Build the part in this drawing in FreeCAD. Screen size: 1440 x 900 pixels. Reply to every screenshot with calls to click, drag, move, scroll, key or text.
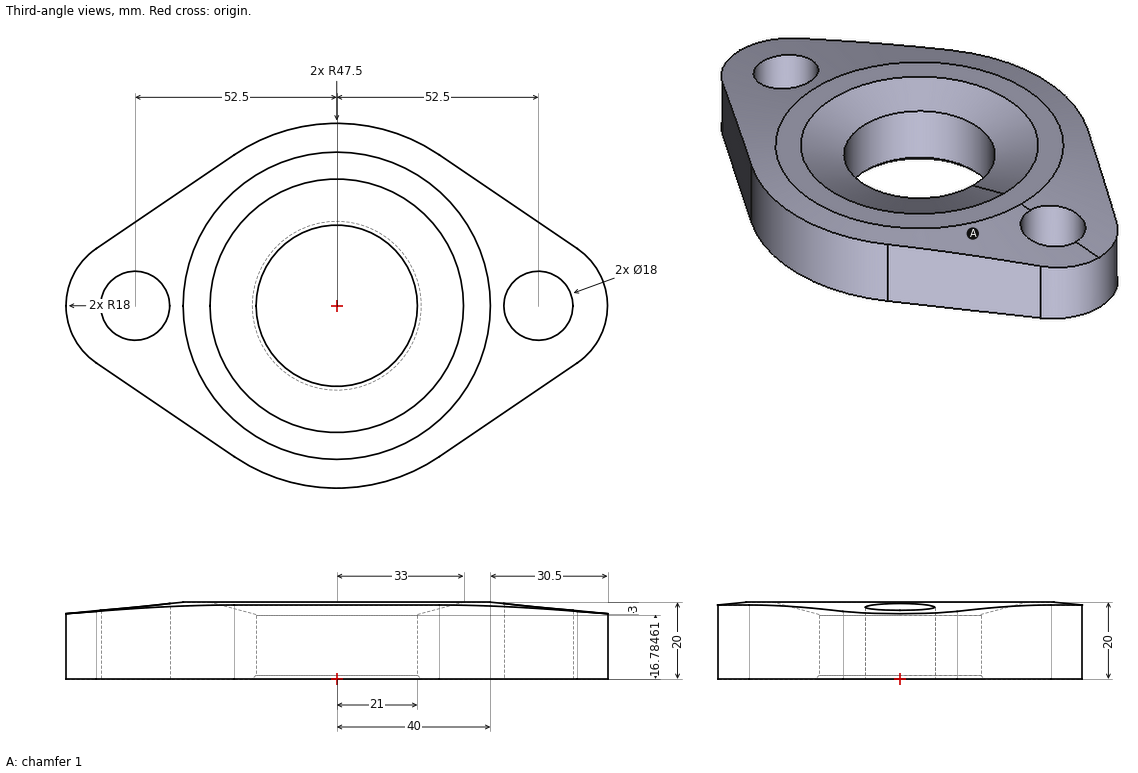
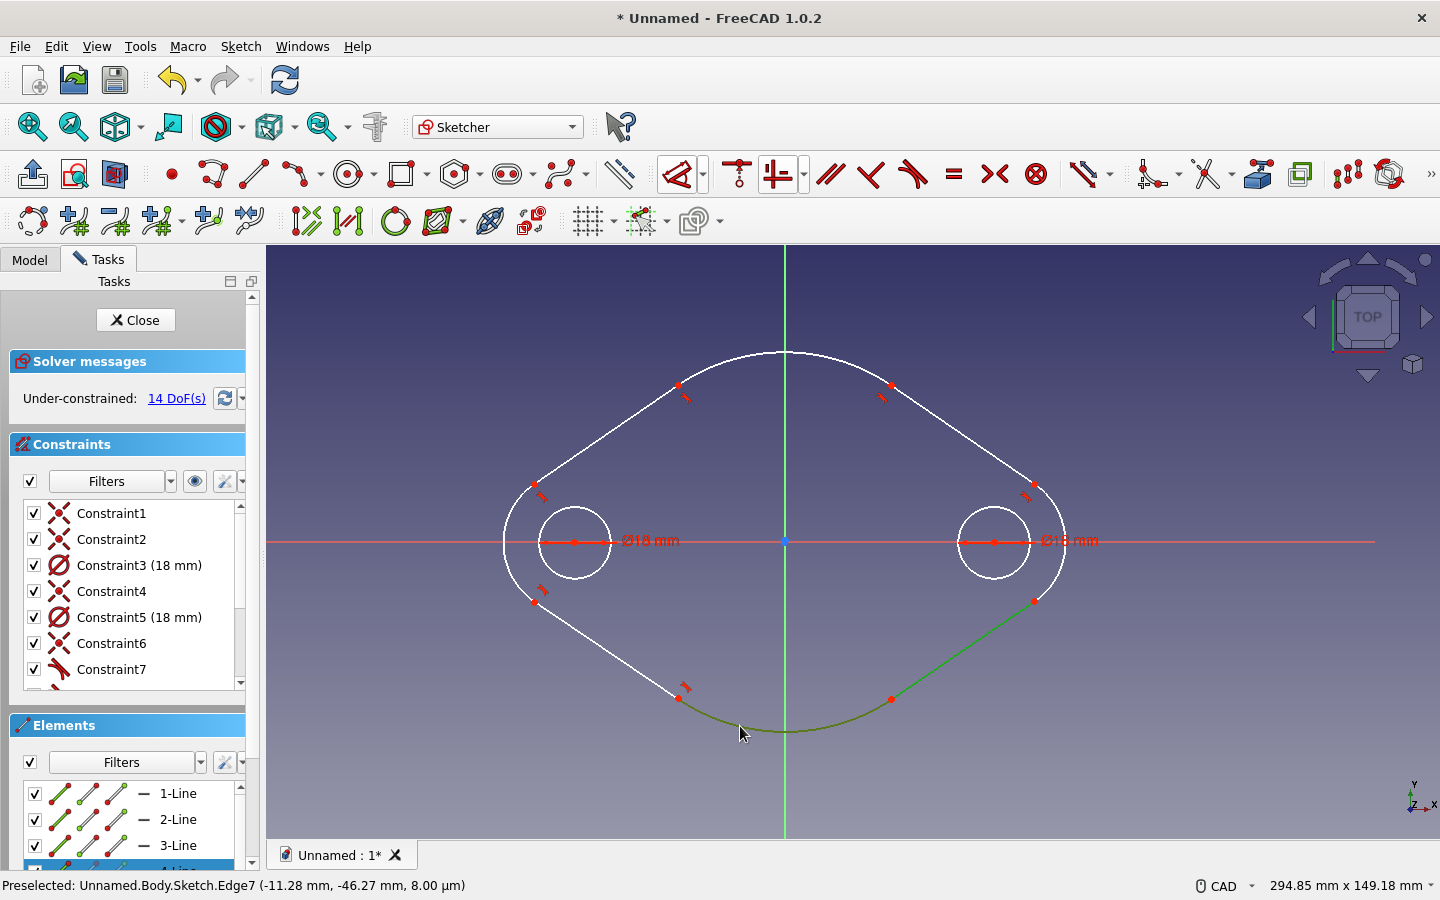
key(t)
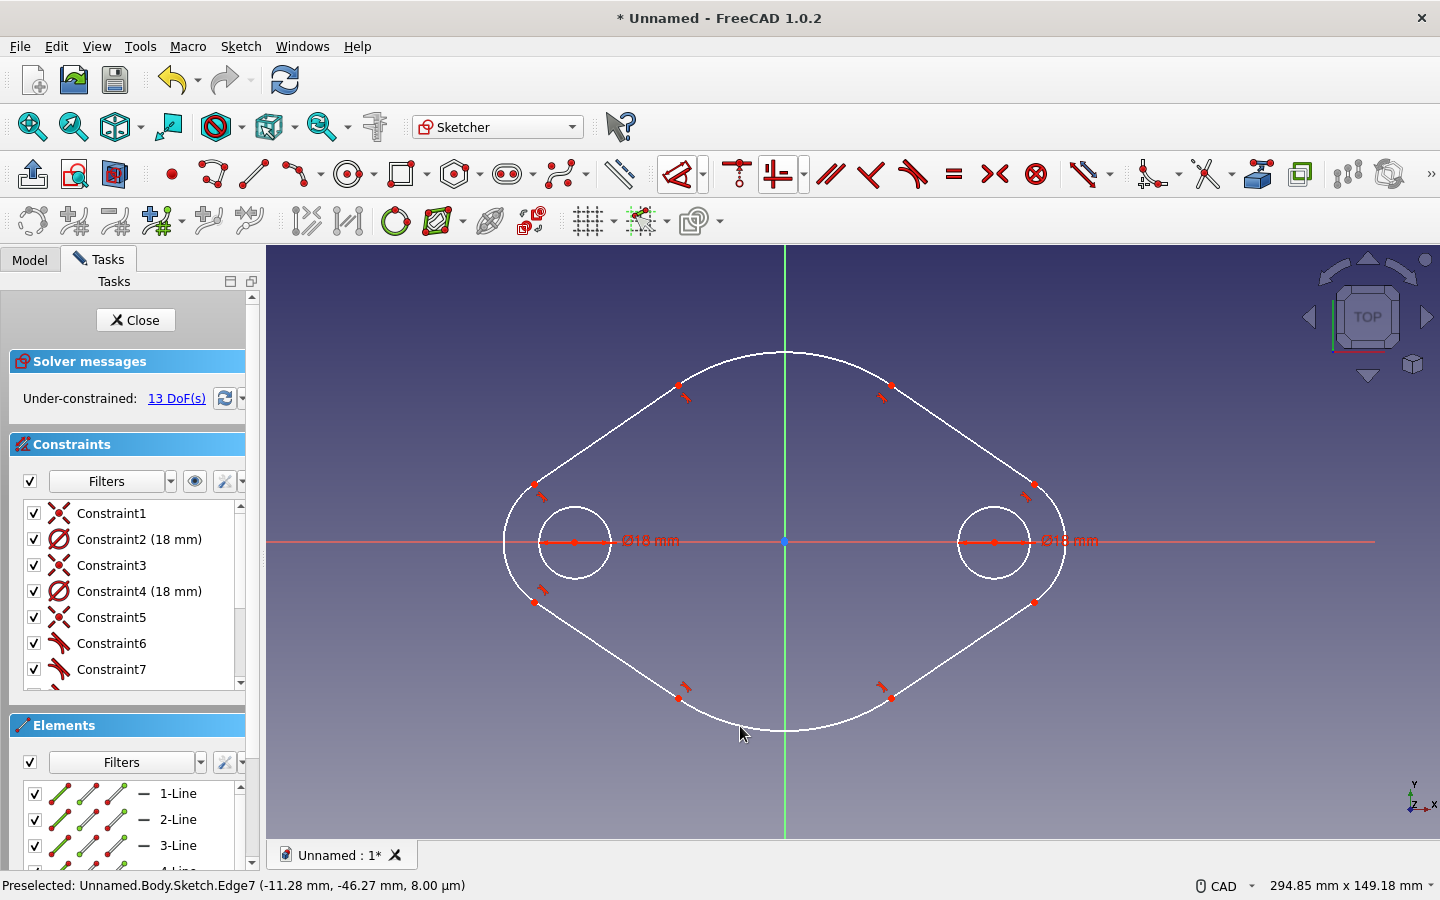
click(934, 670)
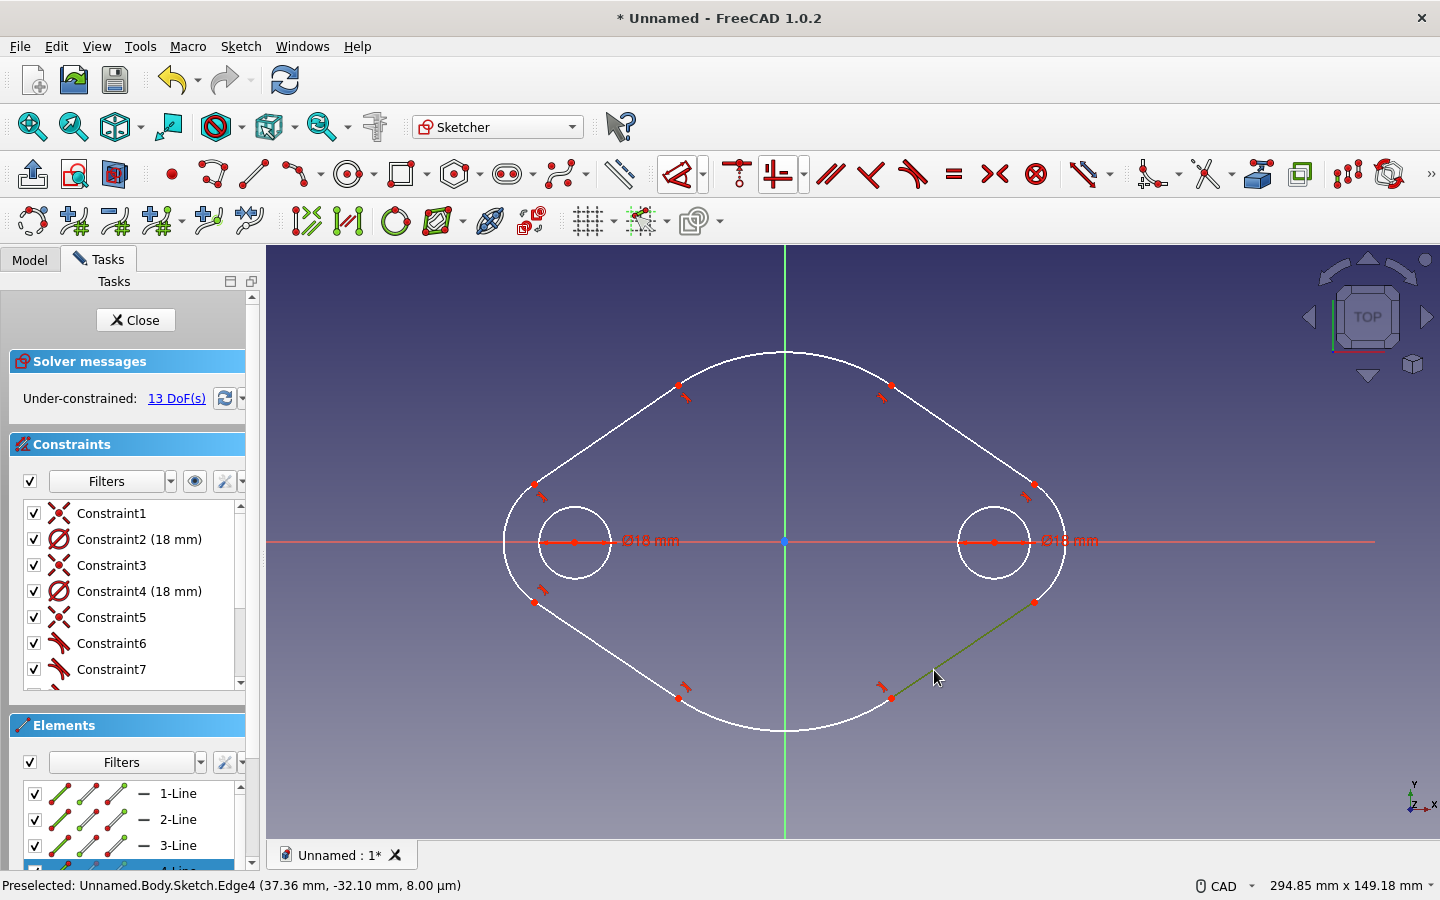
click(1060, 570)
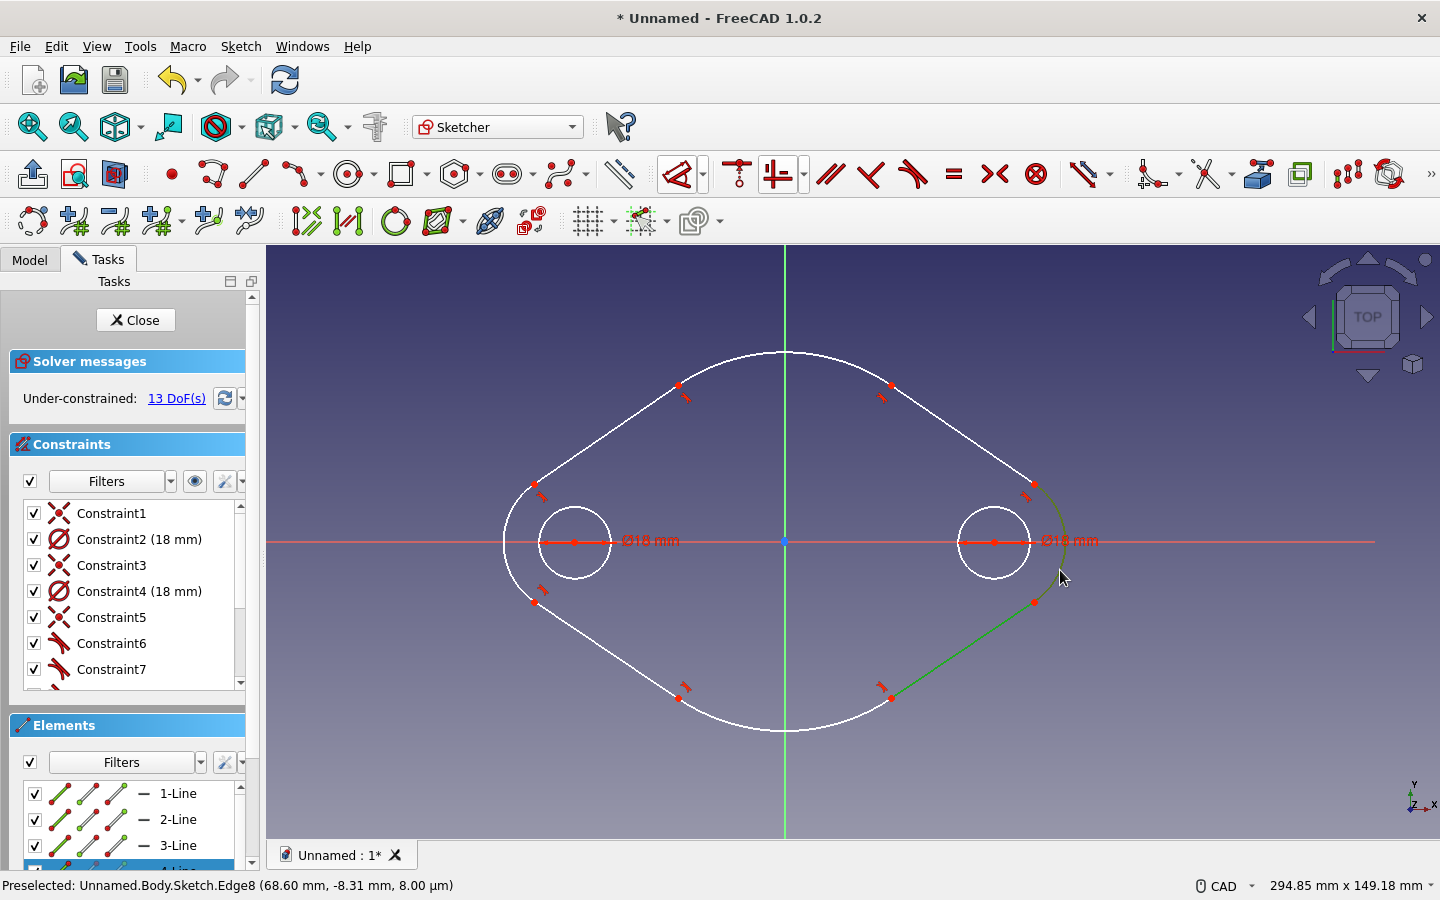
key(t)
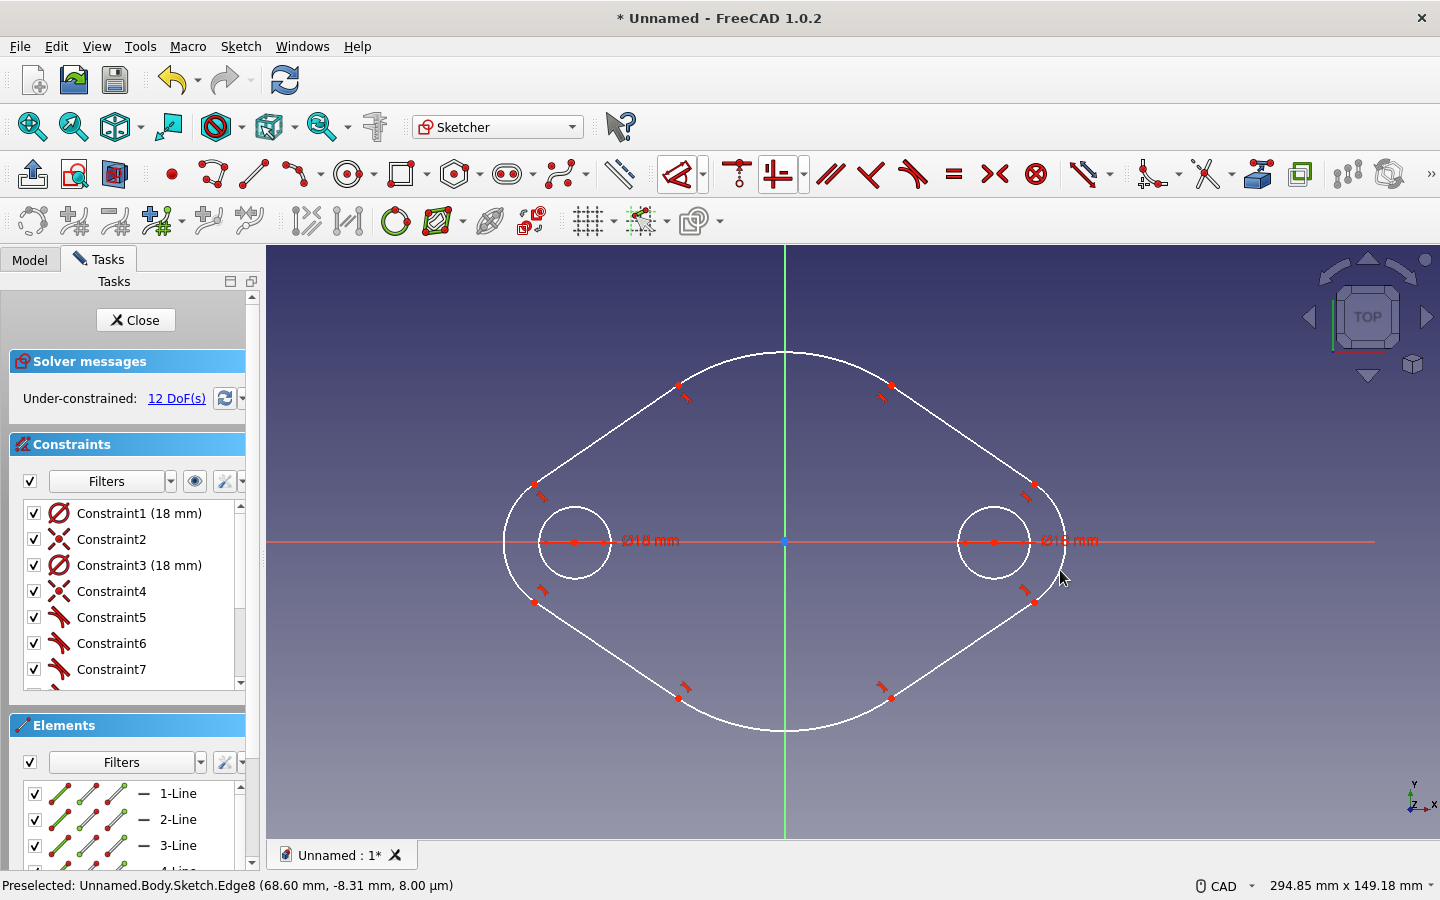
click(829, 358)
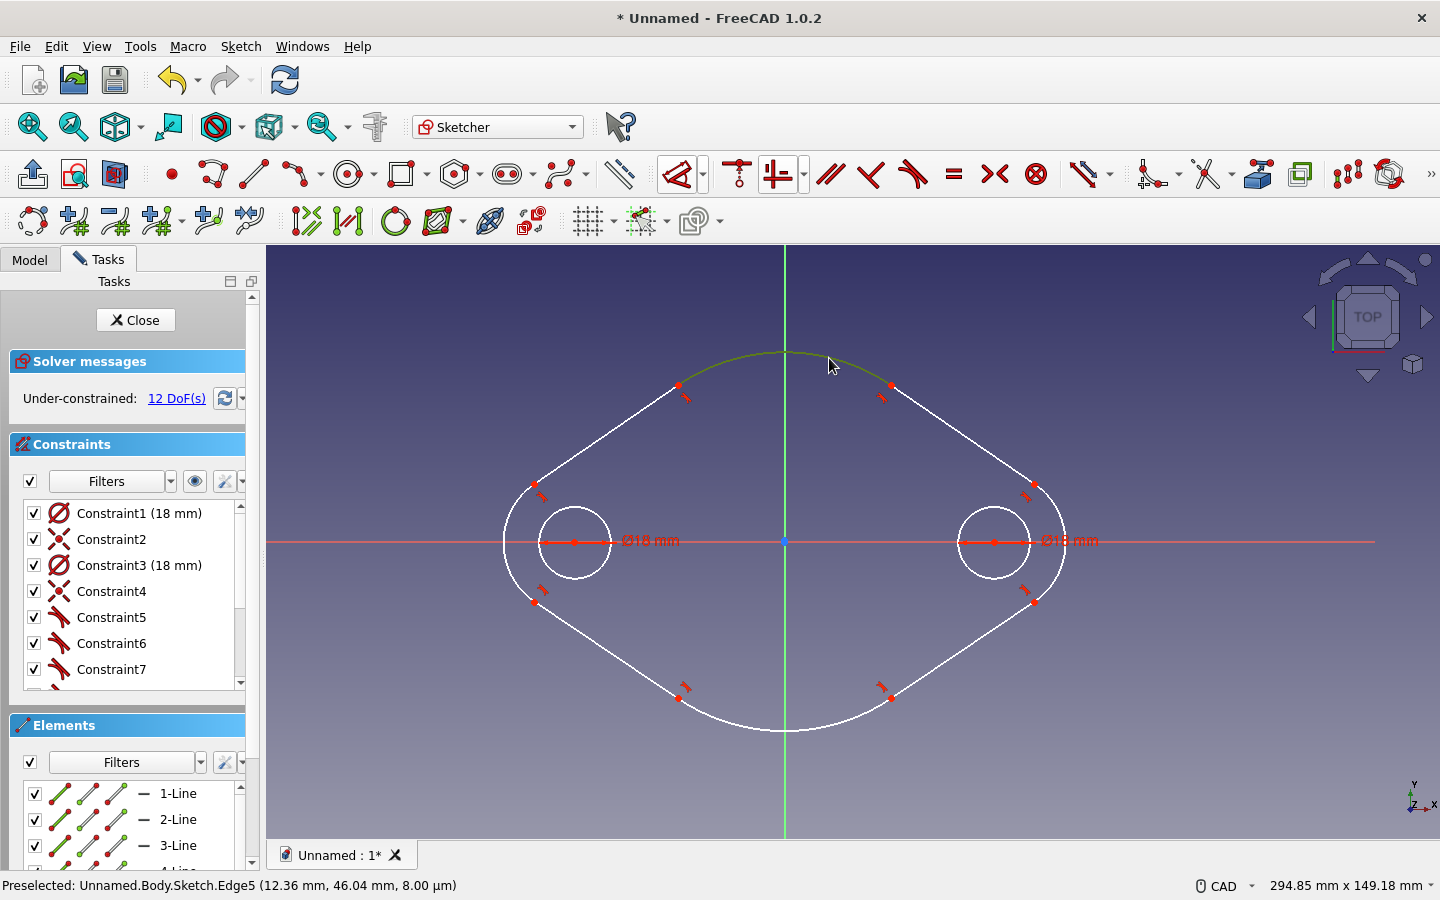
click(740, 726)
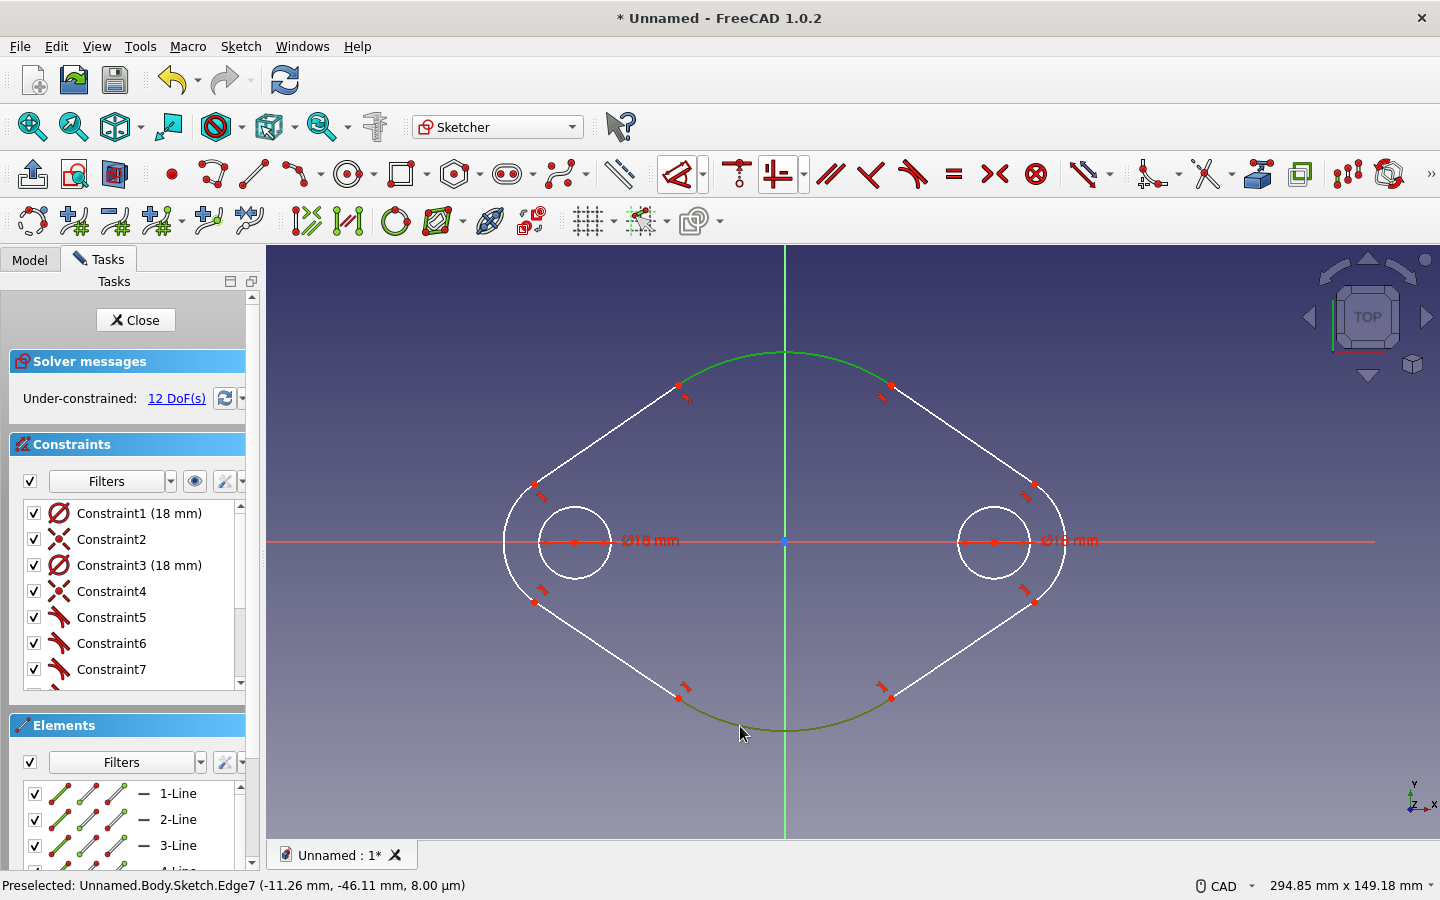
key(c)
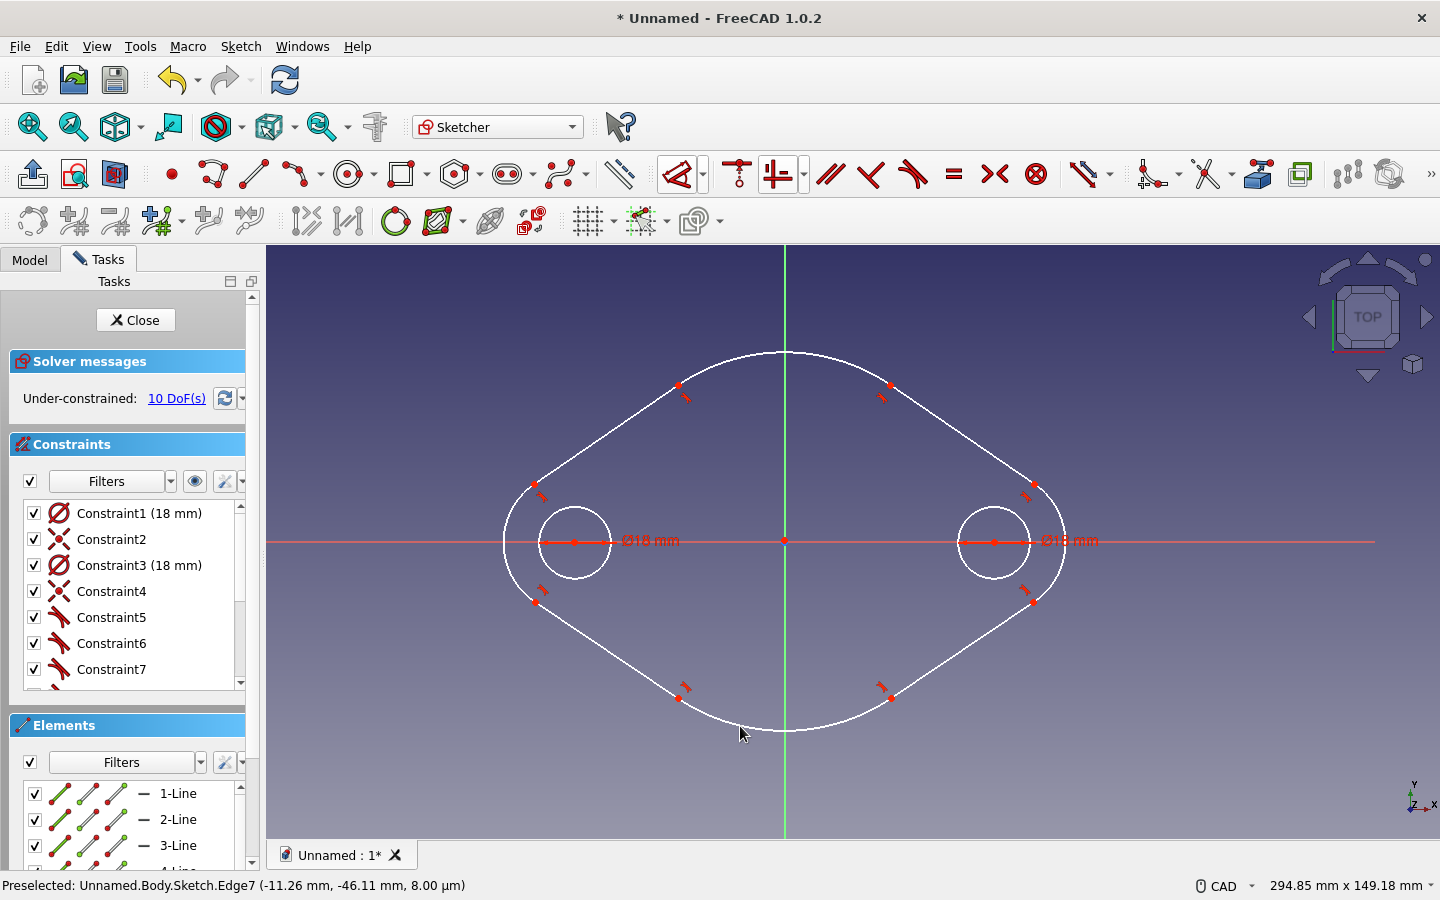
drag(775, 530, 795, 552)